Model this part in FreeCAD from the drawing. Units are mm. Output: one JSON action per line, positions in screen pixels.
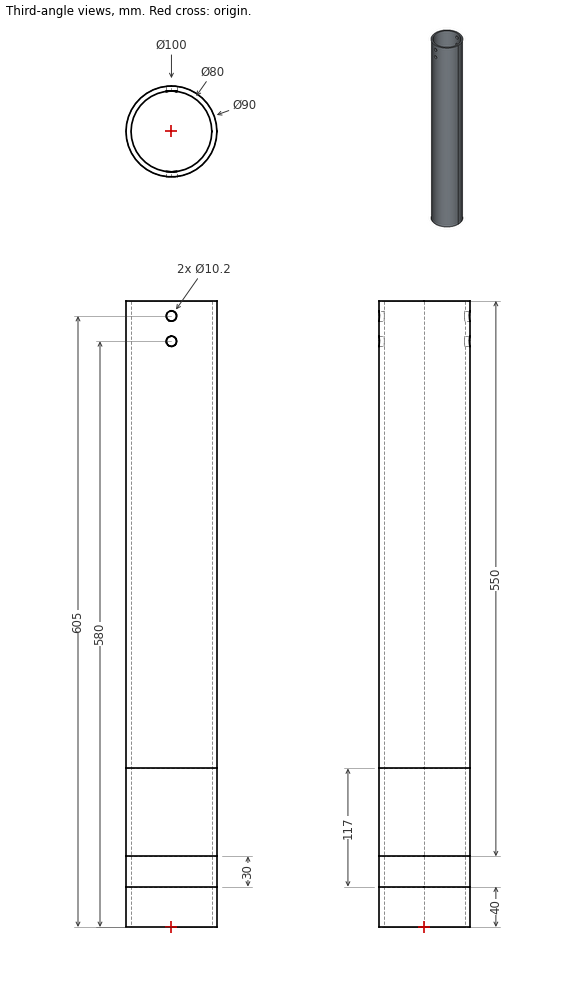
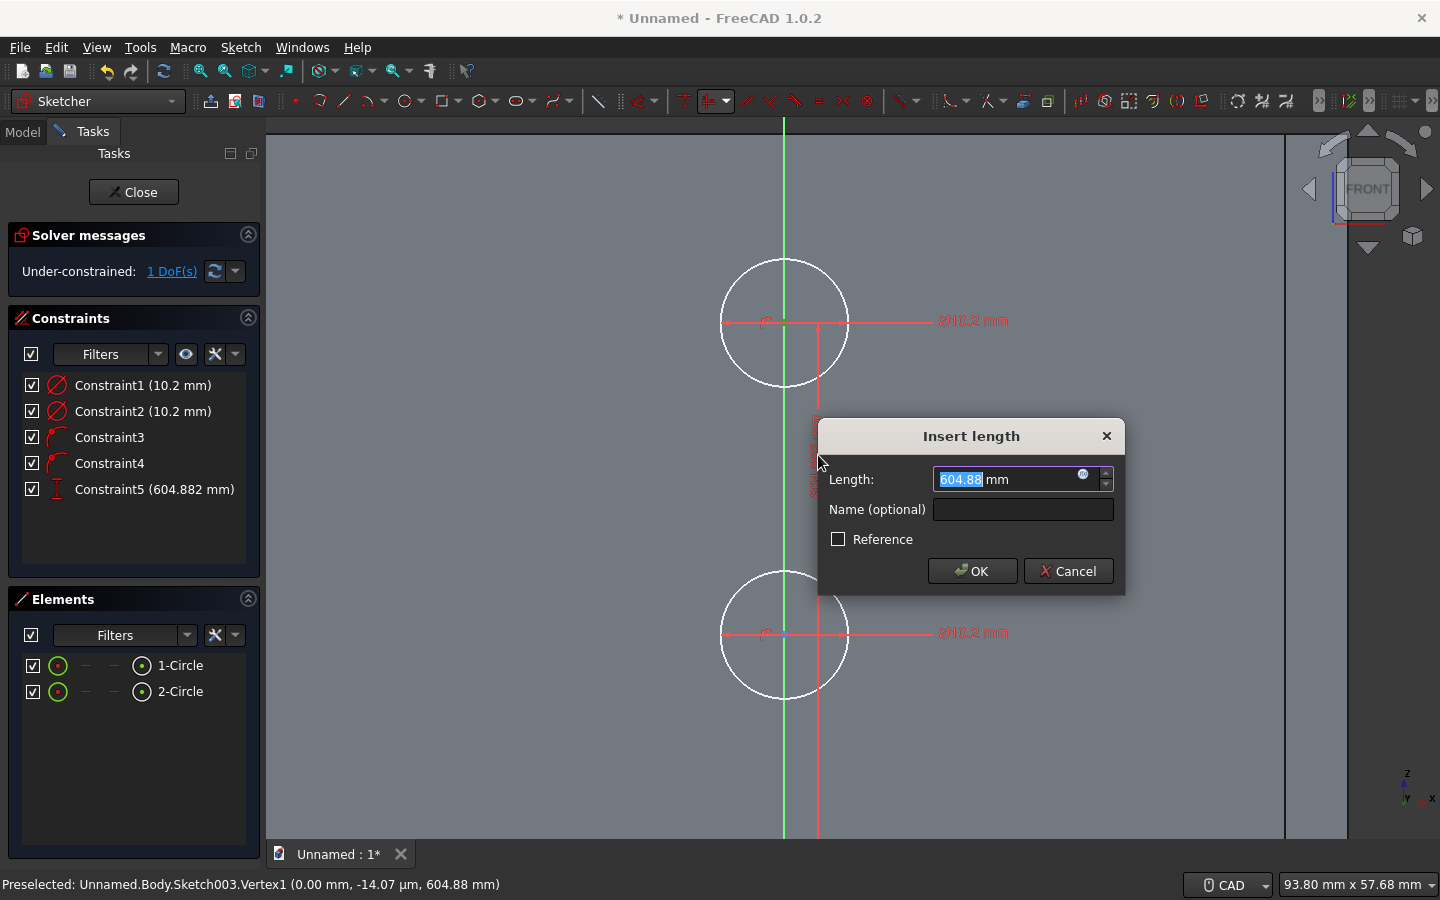
{"action": "type", "text": "605"}
{"action": "key", "text": "Return"}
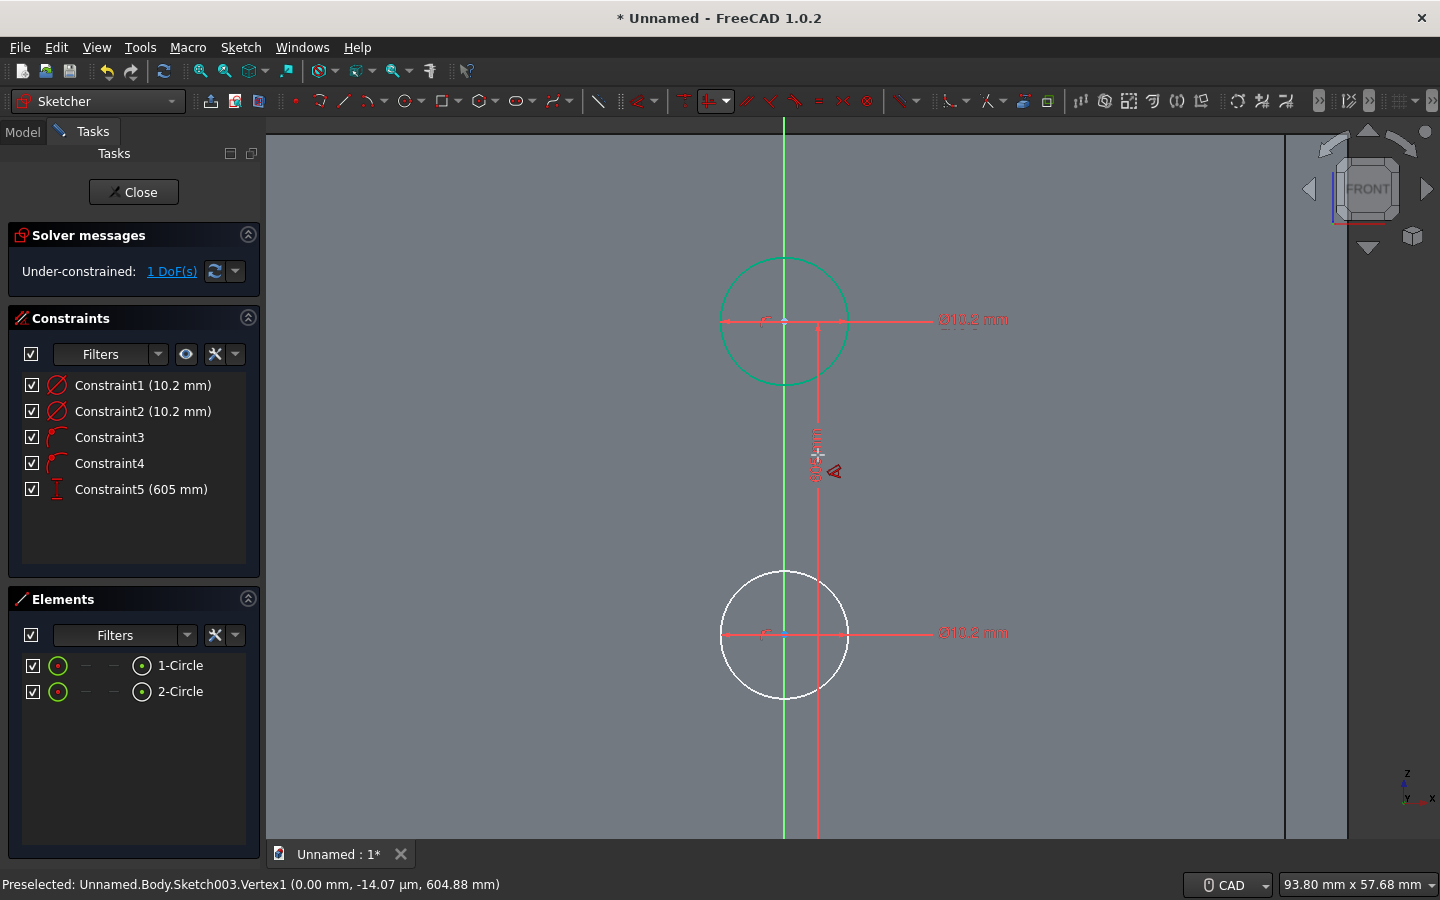
{"action": "left_click", "coordinate": [784, 635]}
{"action": "left_click", "coordinate": [818, 723]}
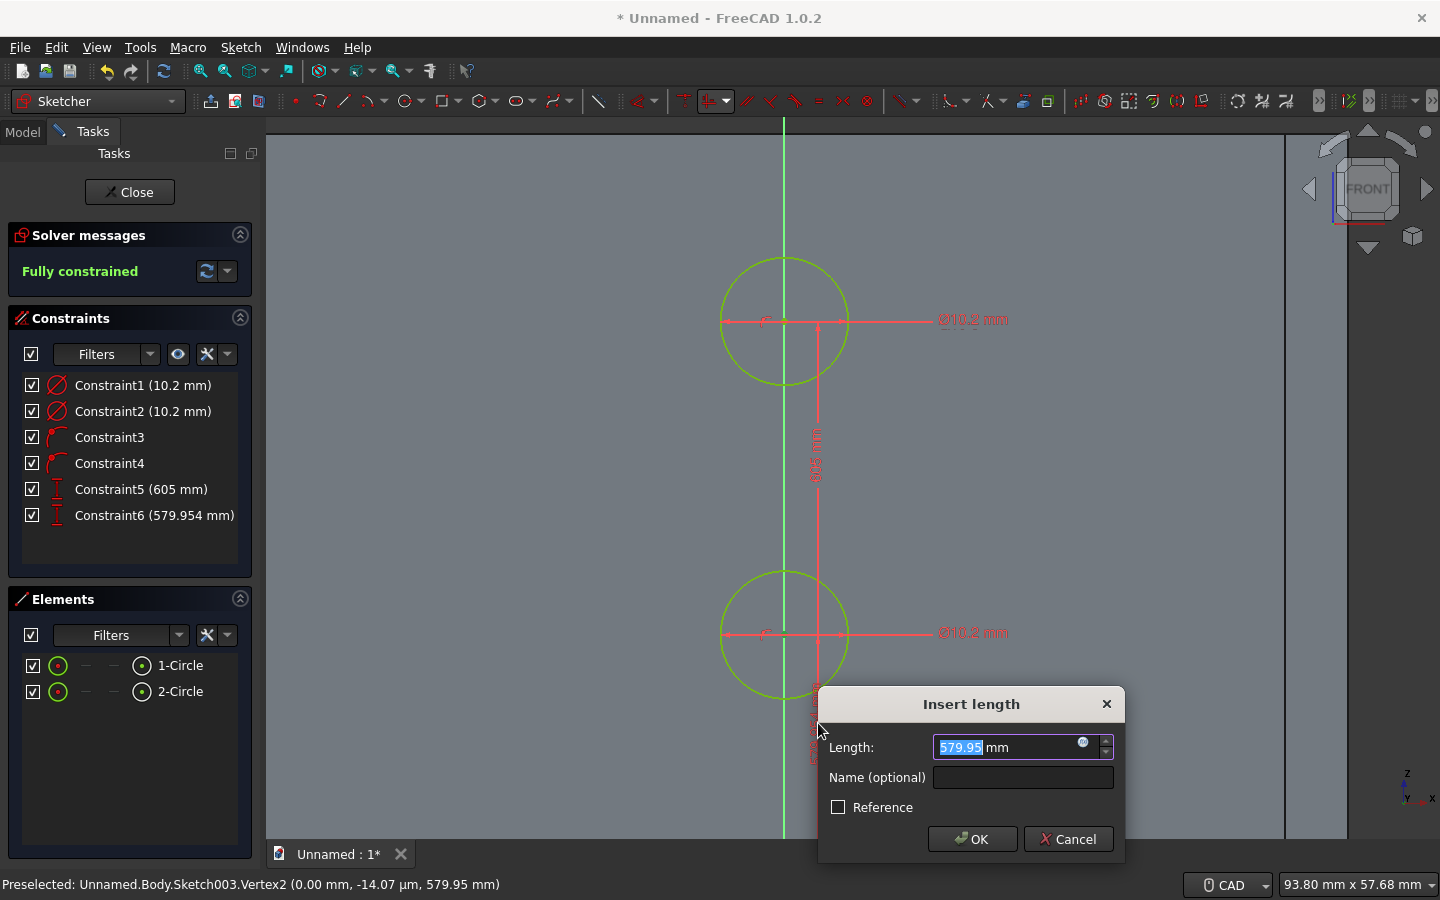
{"action": "type", "text": "580"}
{"action": "key", "text": "Return"}
{"action": "key", "text": "Escape"}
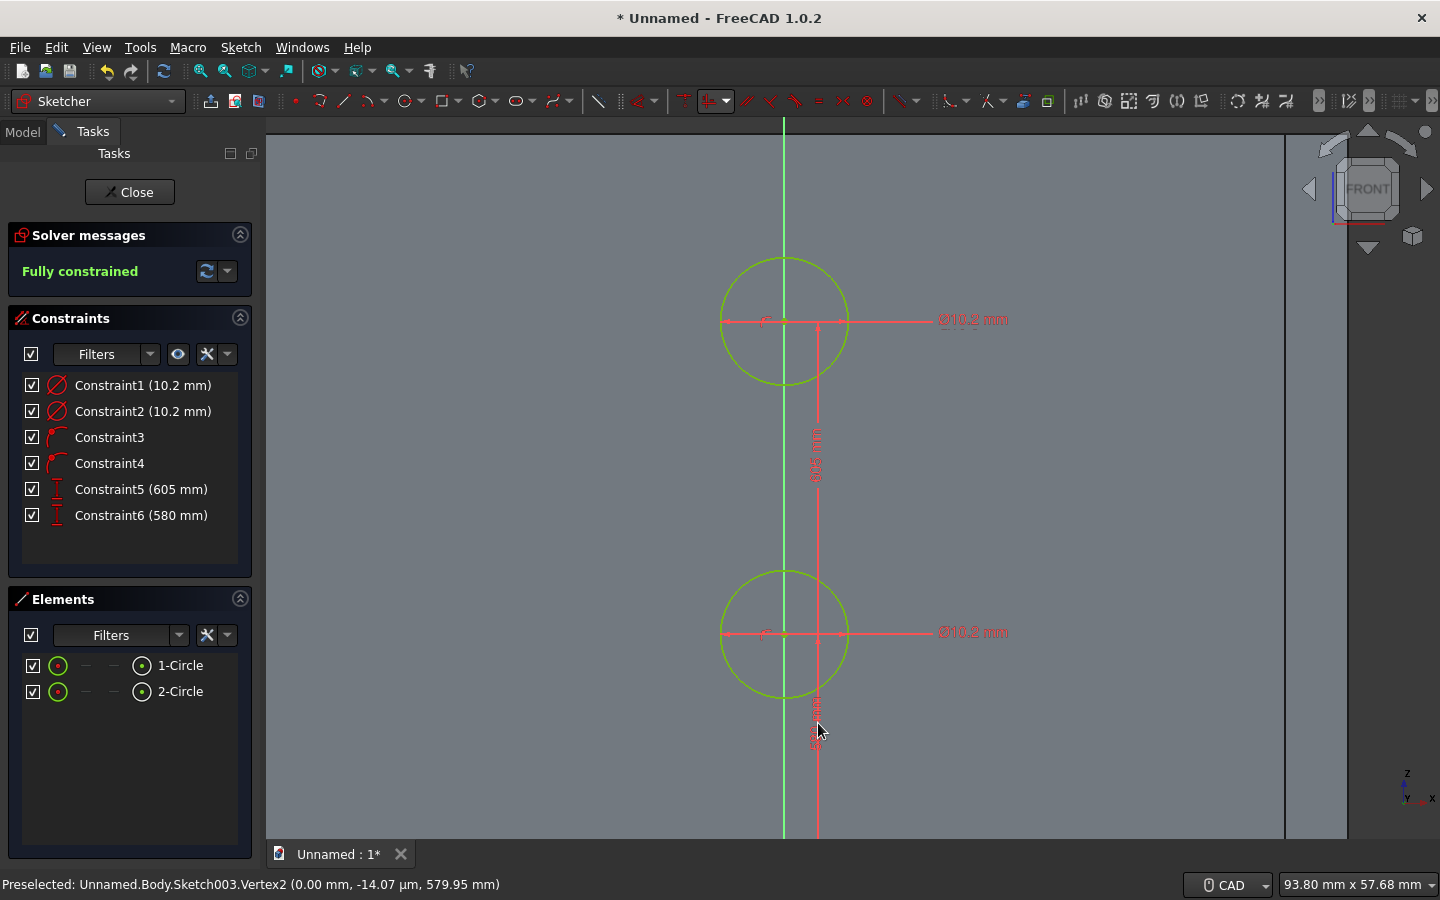
{"action": "left_click", "coordinate": [130, 192]}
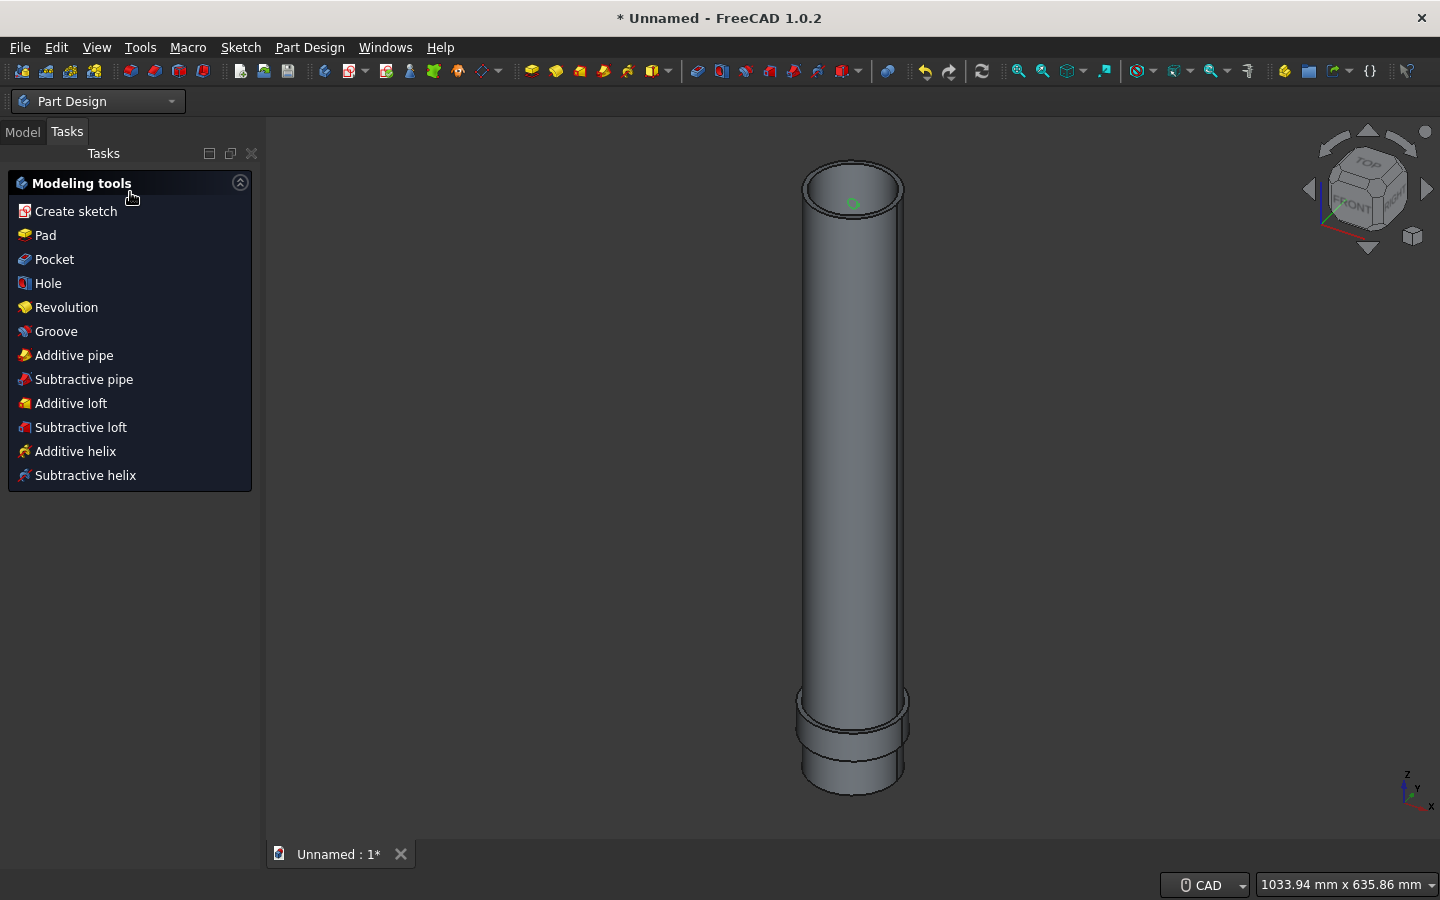
{"action": "left_click", "coordinate": [698, 72]}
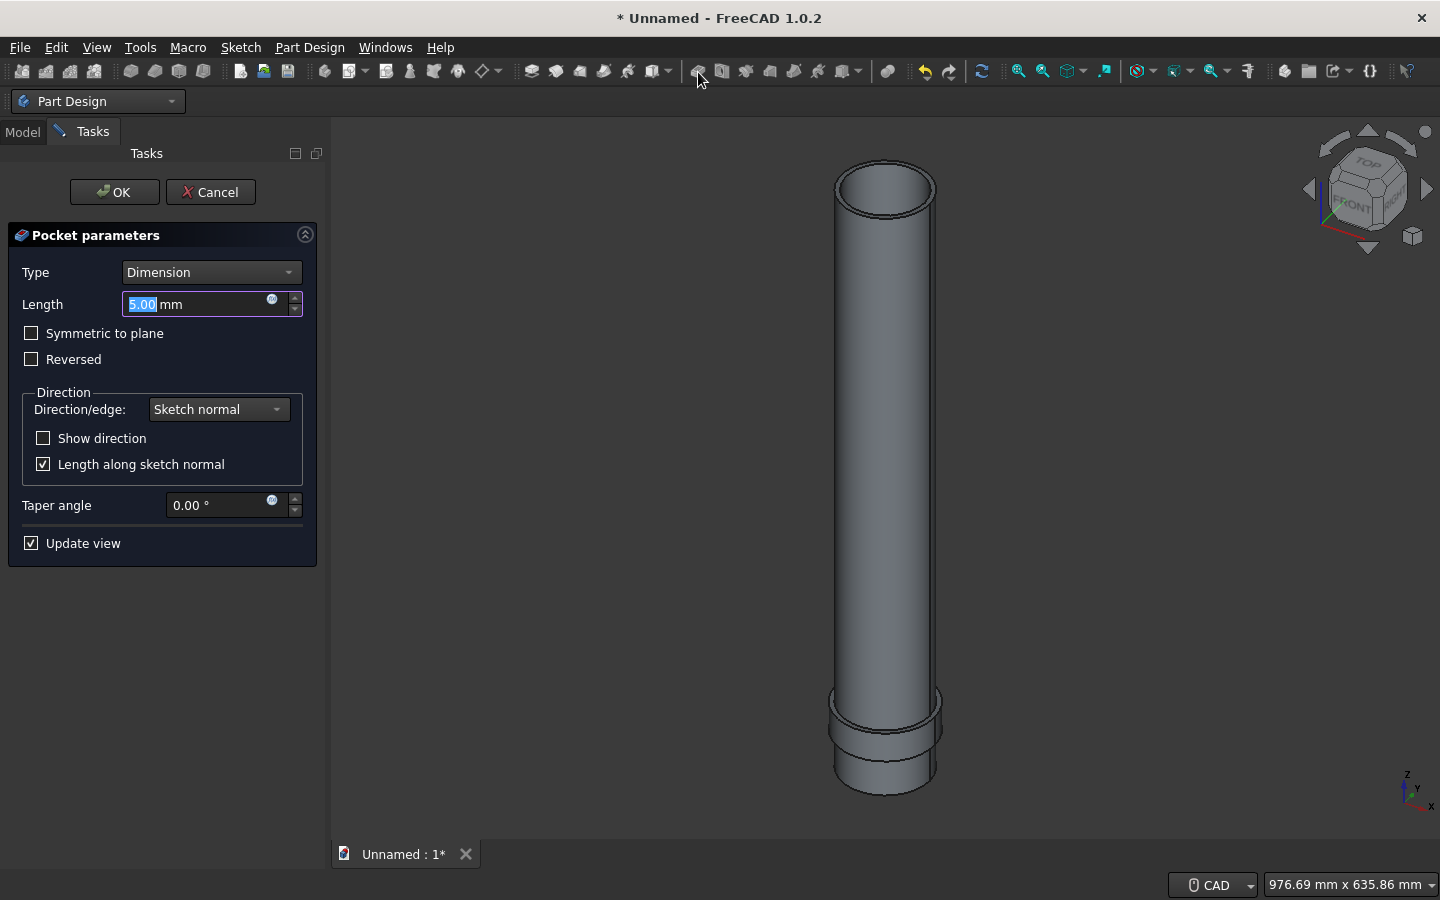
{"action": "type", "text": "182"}
{"action": "key", "text": "Tab"}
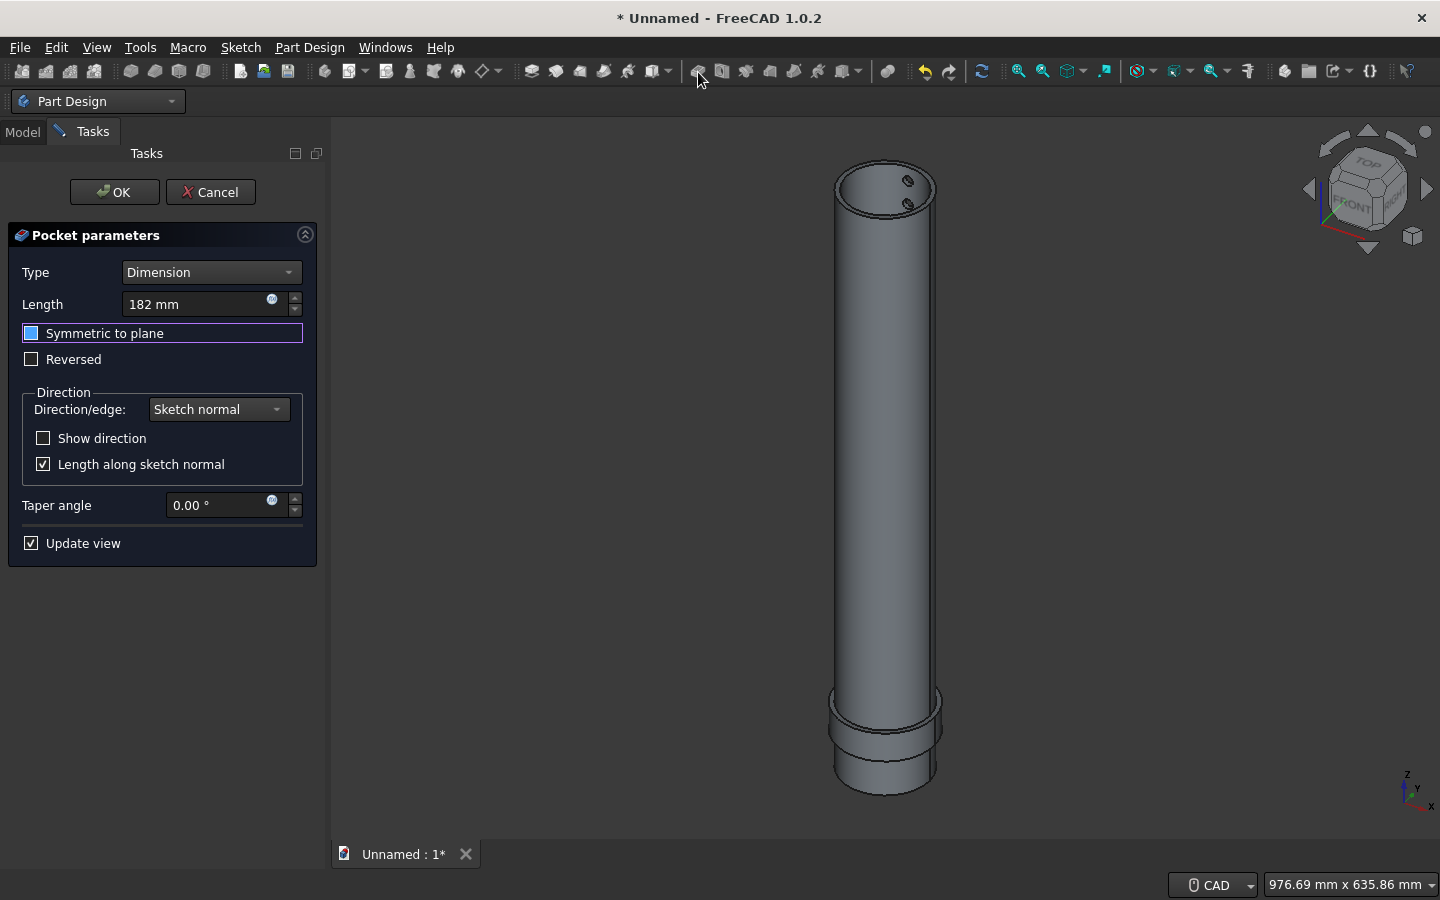
{"action": "left_click", "coordinate": [30, 333]}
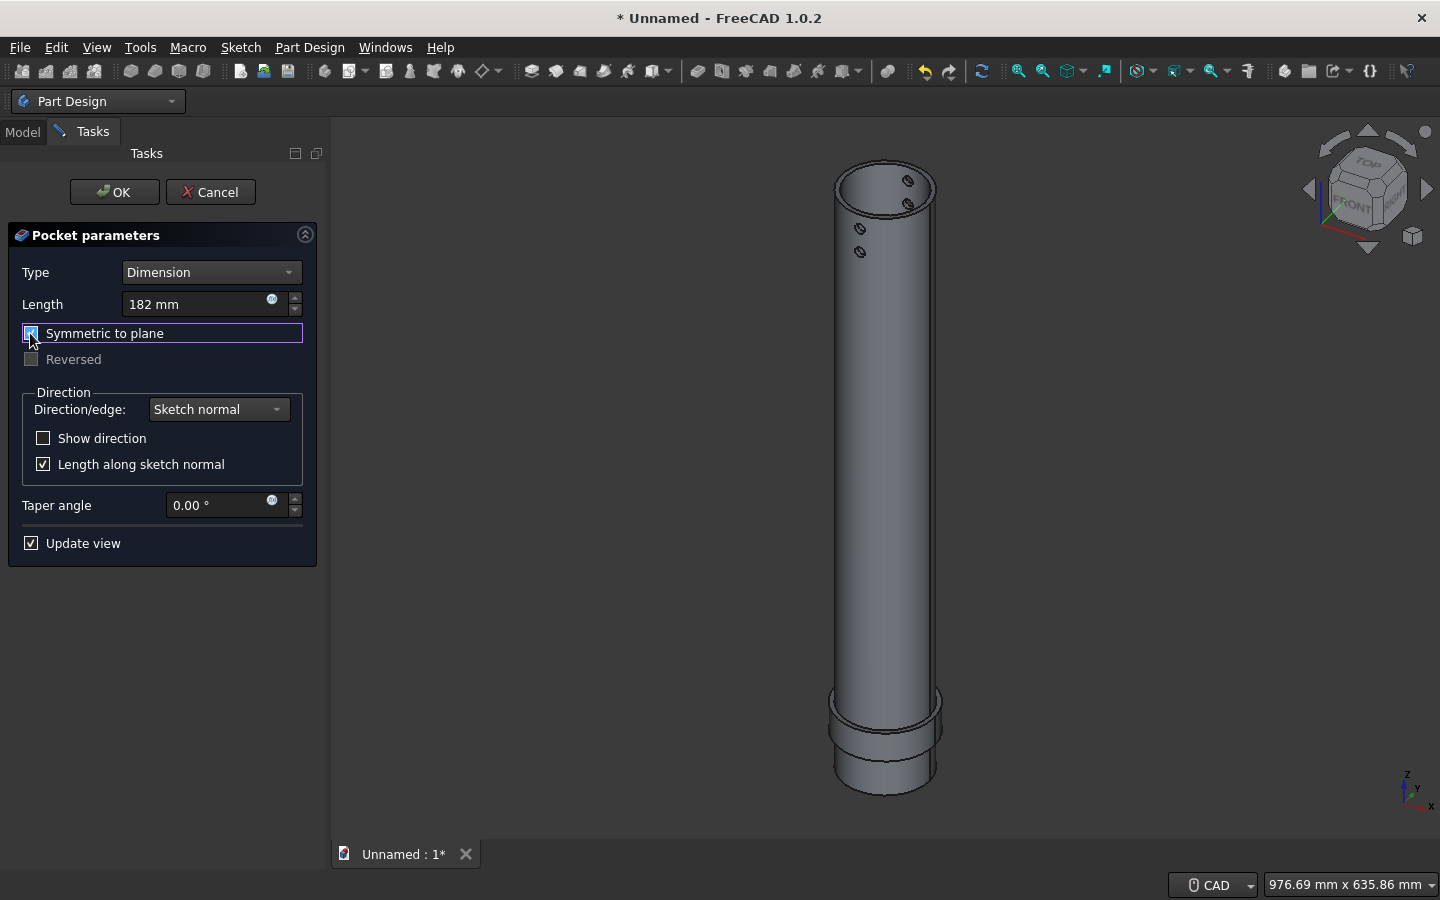
{"action": "left_click", "coordinate": [115, 192]}